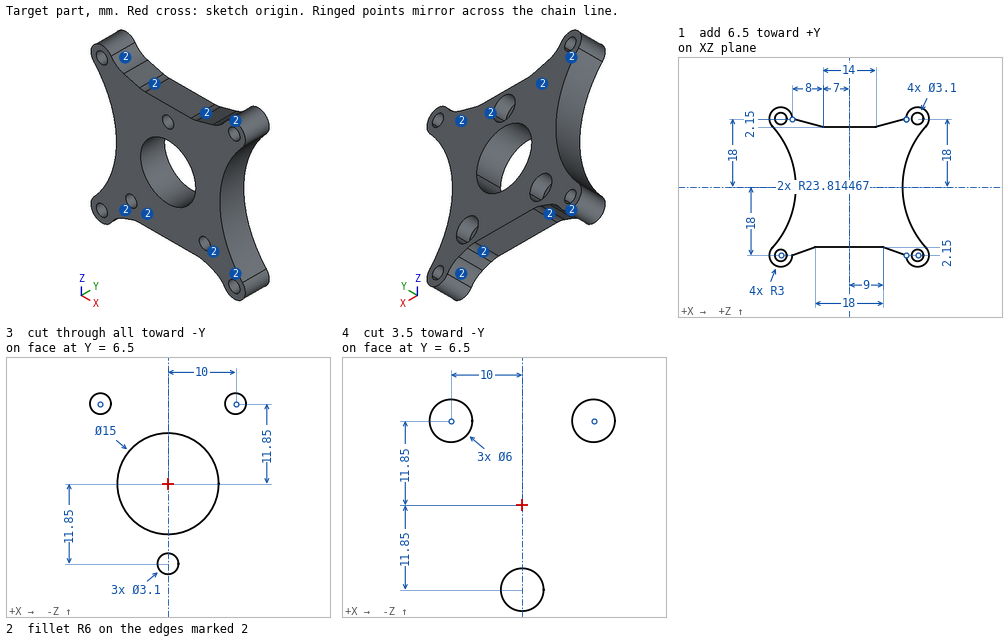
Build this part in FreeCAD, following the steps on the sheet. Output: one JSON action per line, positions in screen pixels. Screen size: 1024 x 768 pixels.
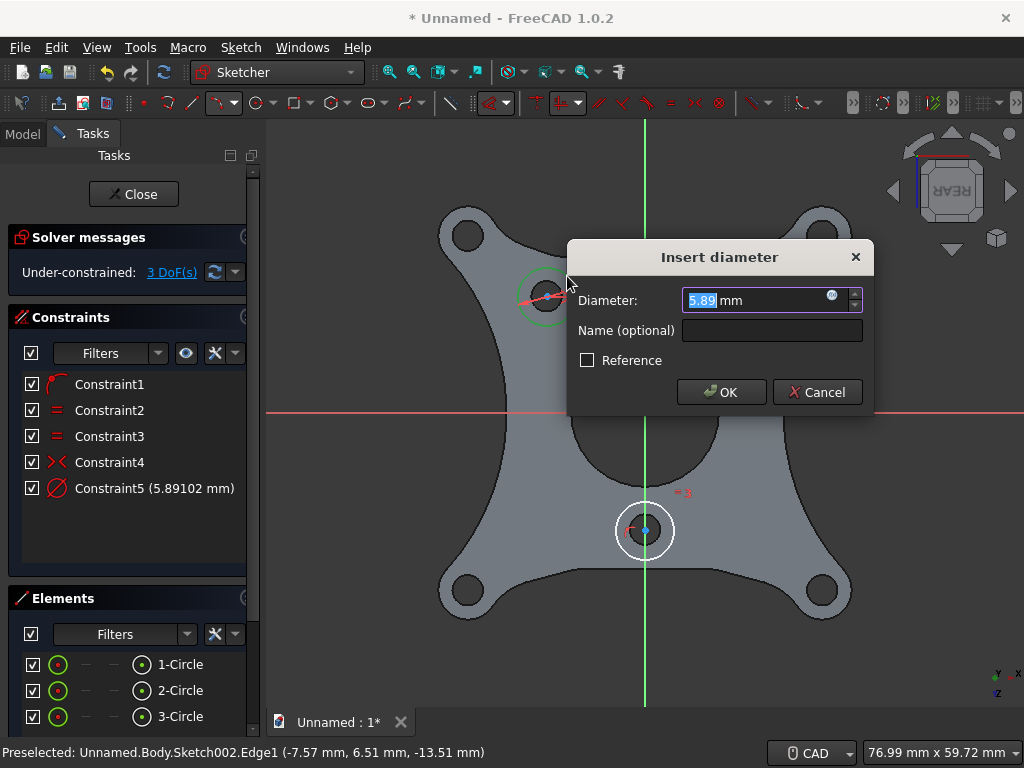
{"action": "type", "text": "6"}
{"action": "key", "text": "Return"}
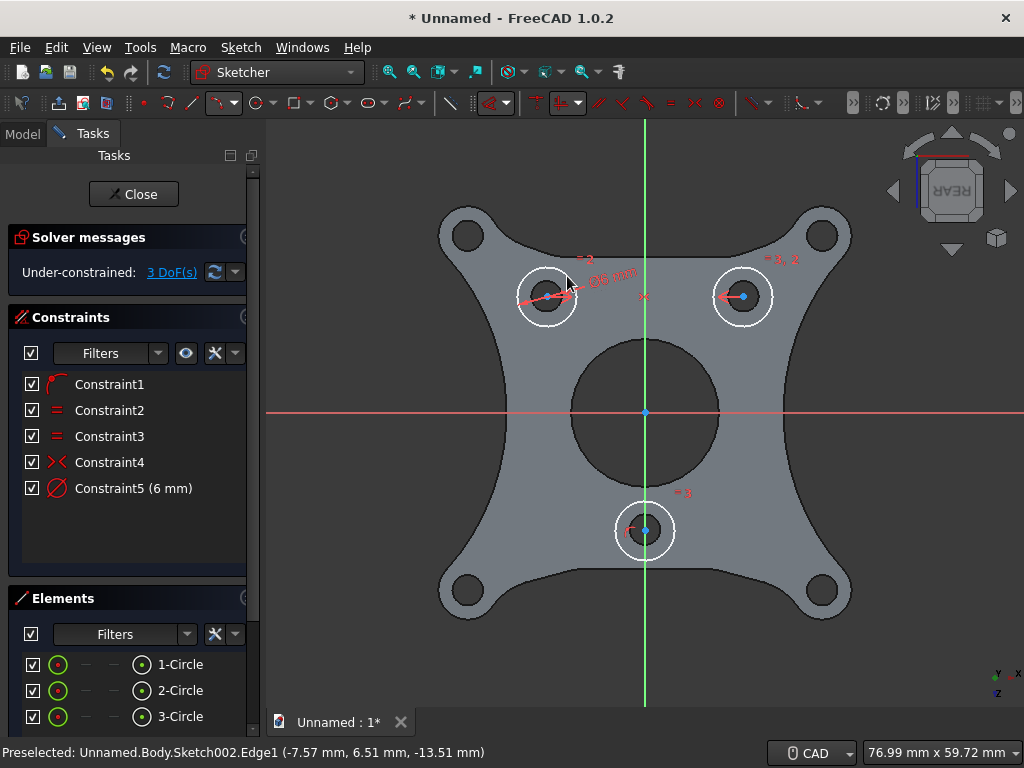
{"action": "left_click", "coordinate": [547, 297]}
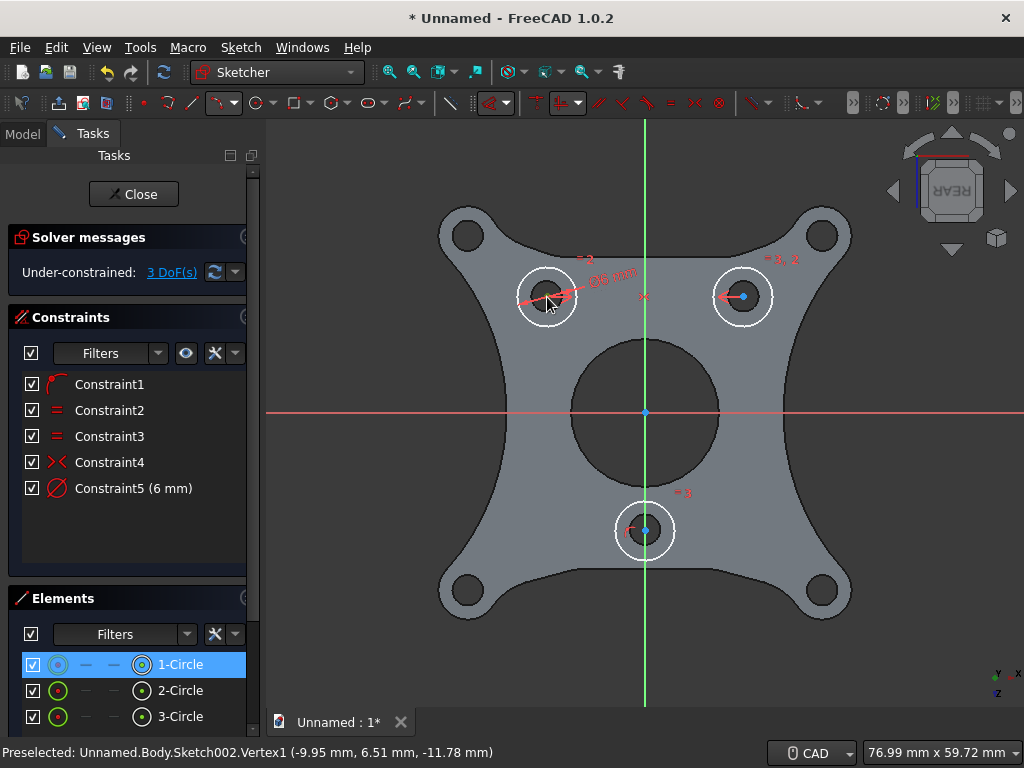
{"action": "left_click", "coordinate": [508, 104]}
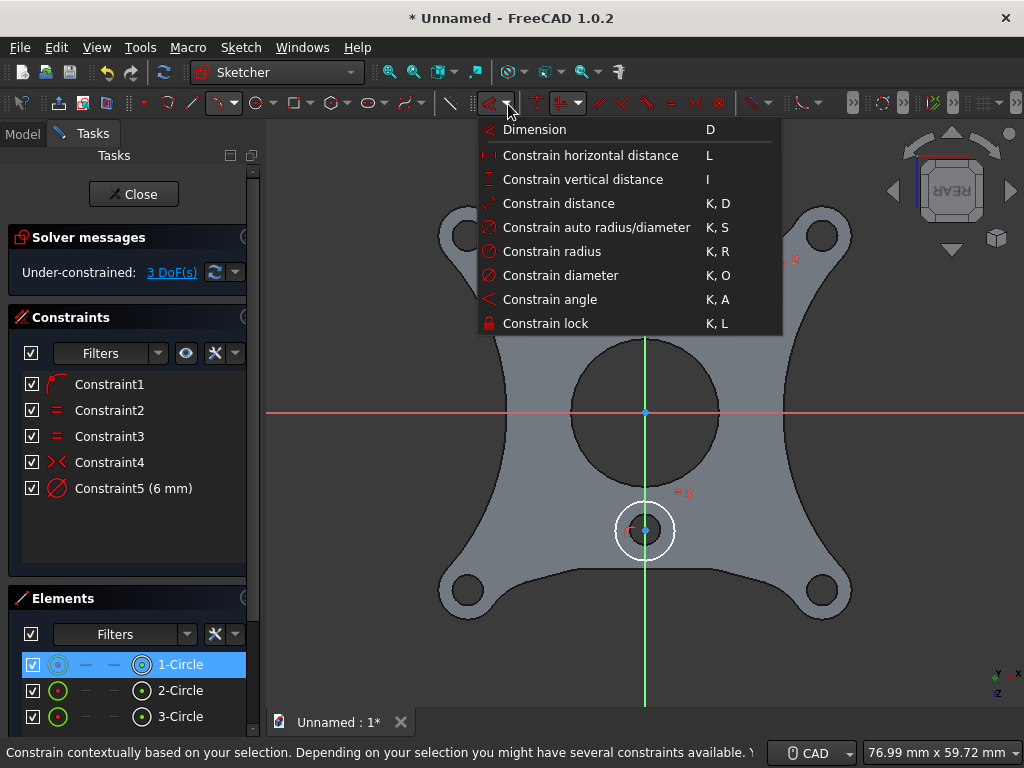
{"action": "left_click", "coordinate": [630, 155]}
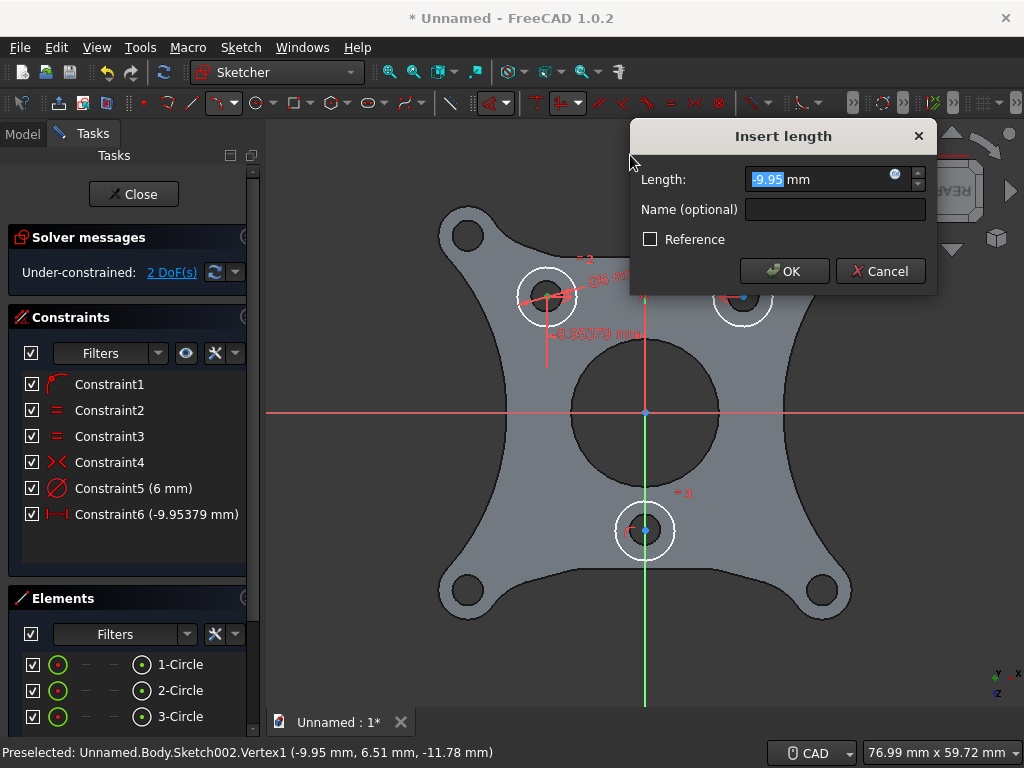
{"action": "type", "text": "-10"}
{"action": "key", "text": "Return"}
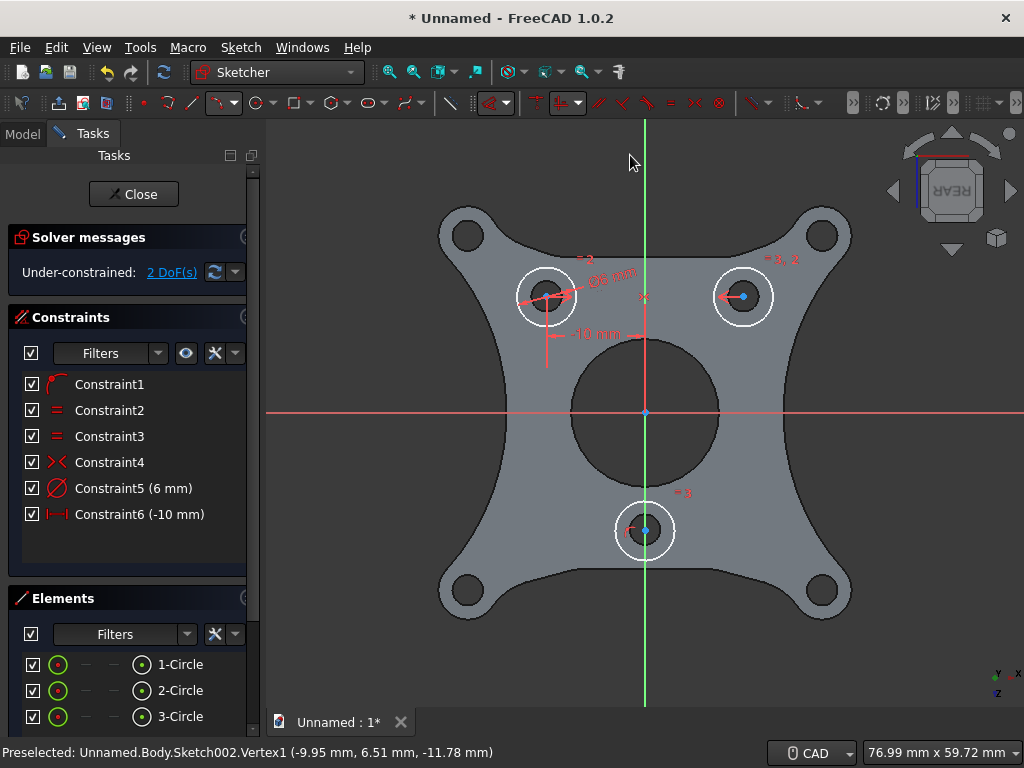
{"action": "left_click", "coordinate": [547, 297]}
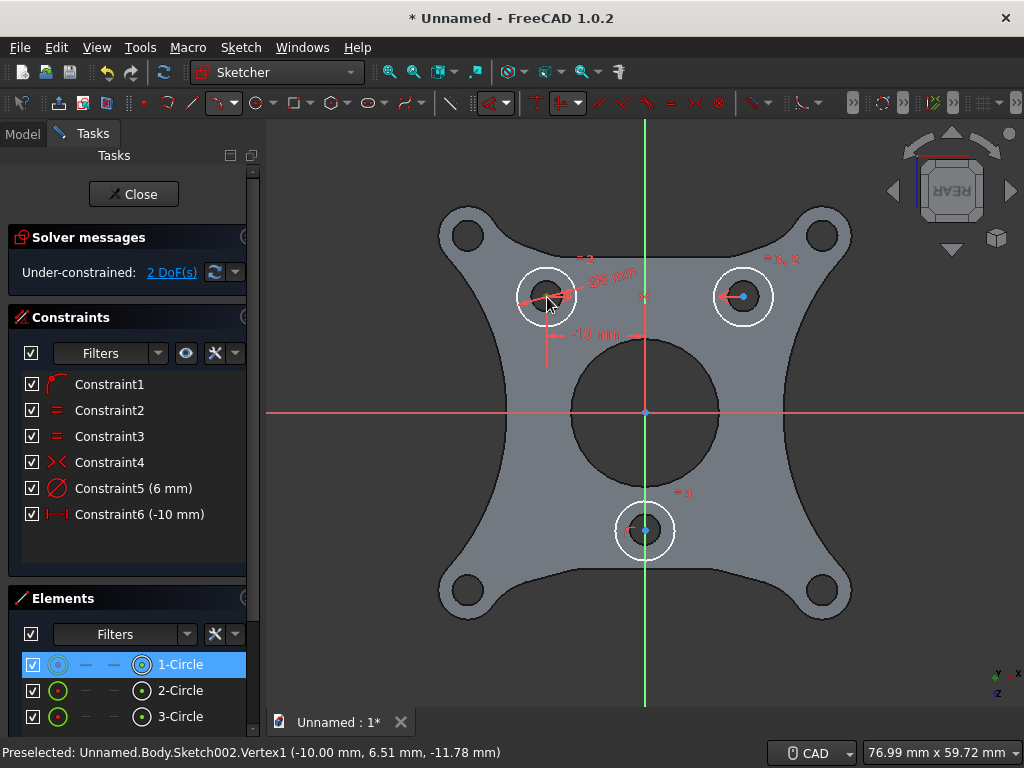
{"action": "left_click", "coordinate": [508, 104]}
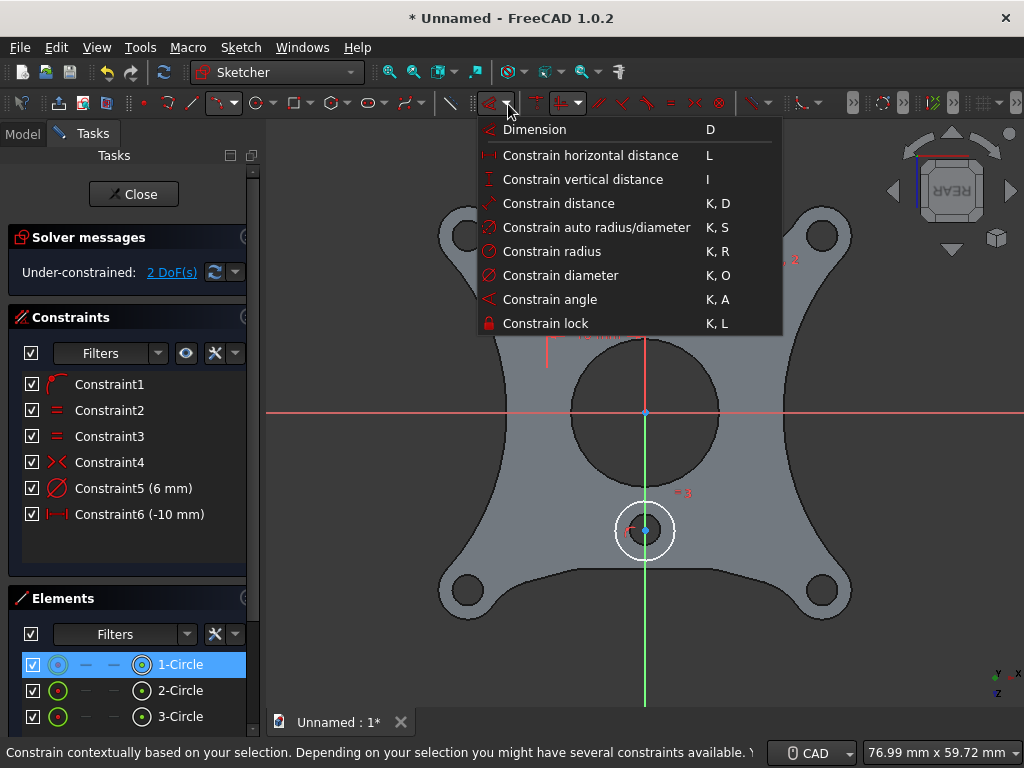
{"action": "left_click", "coordinate": [630, 179]}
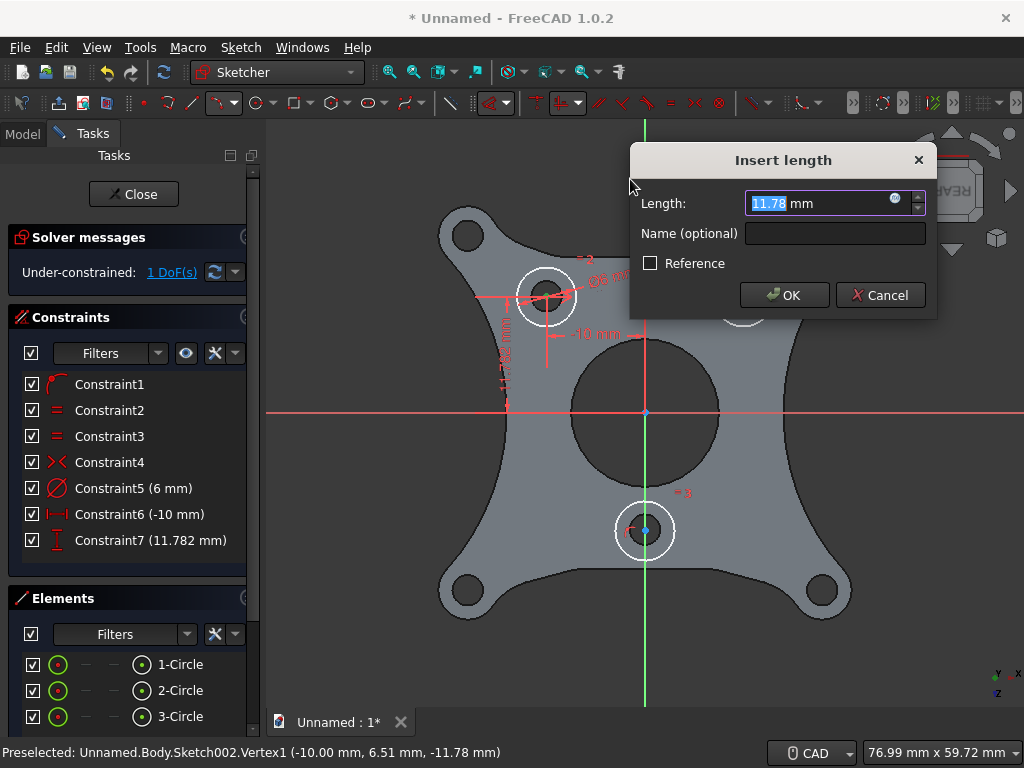
{"action": "type", "text": "11.85"}
{"action": "key", "text": "Return"}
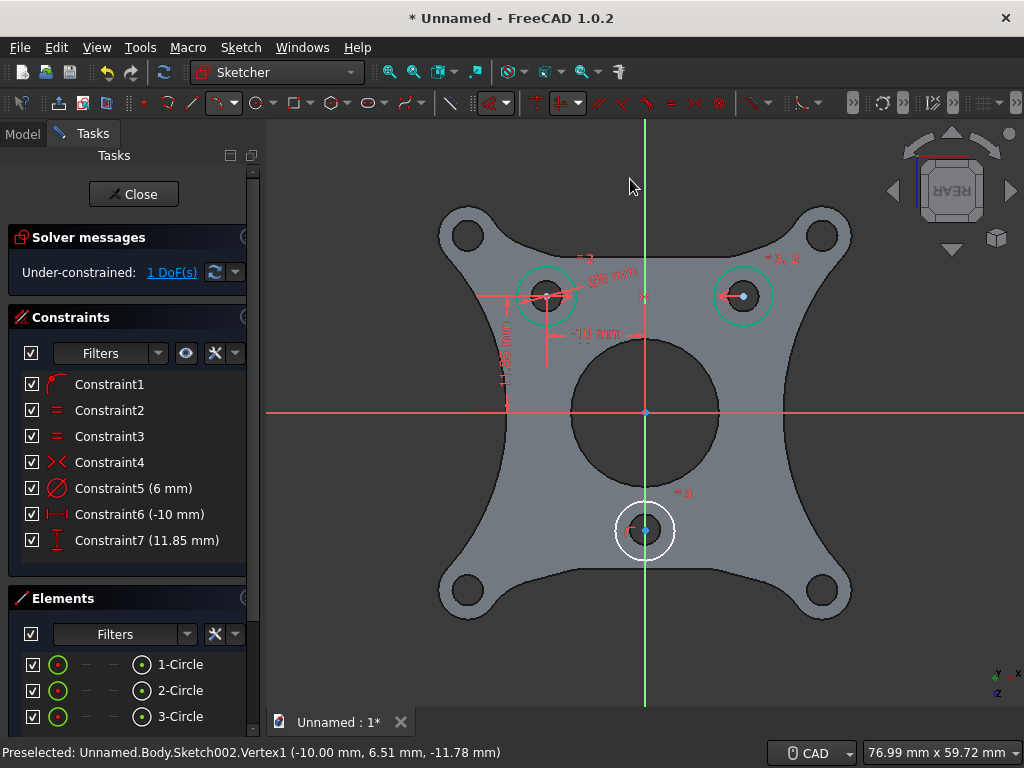
{"action": "left_click", "coordinate": [645, 531]}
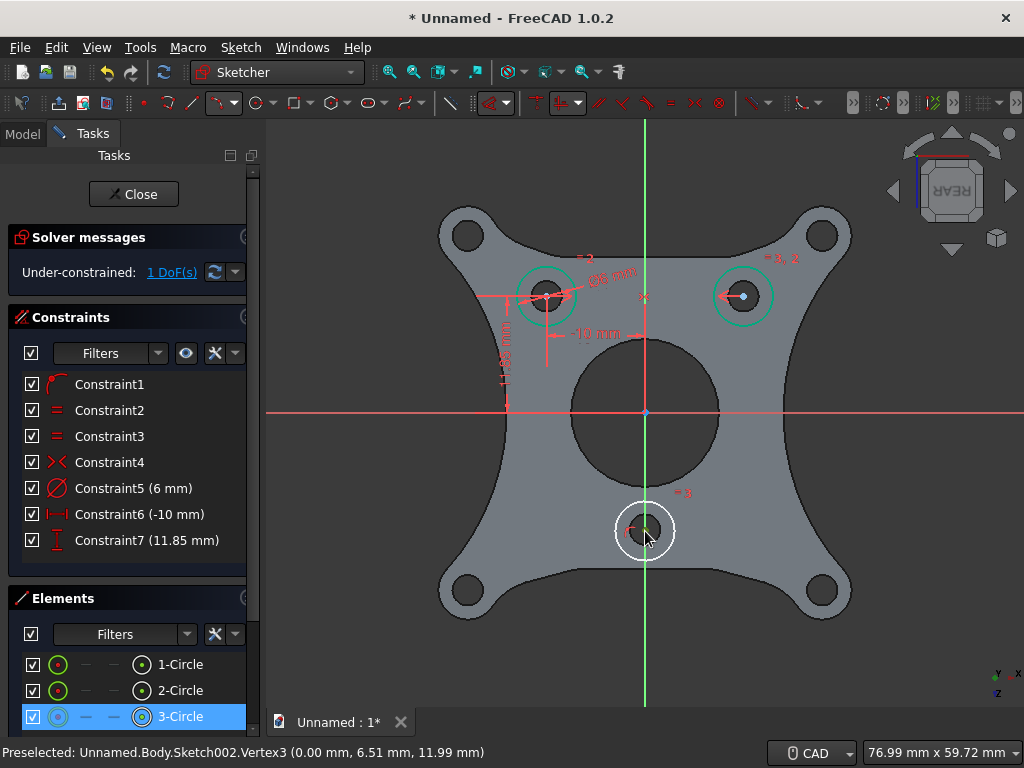
{"action": "key", "text": "i"}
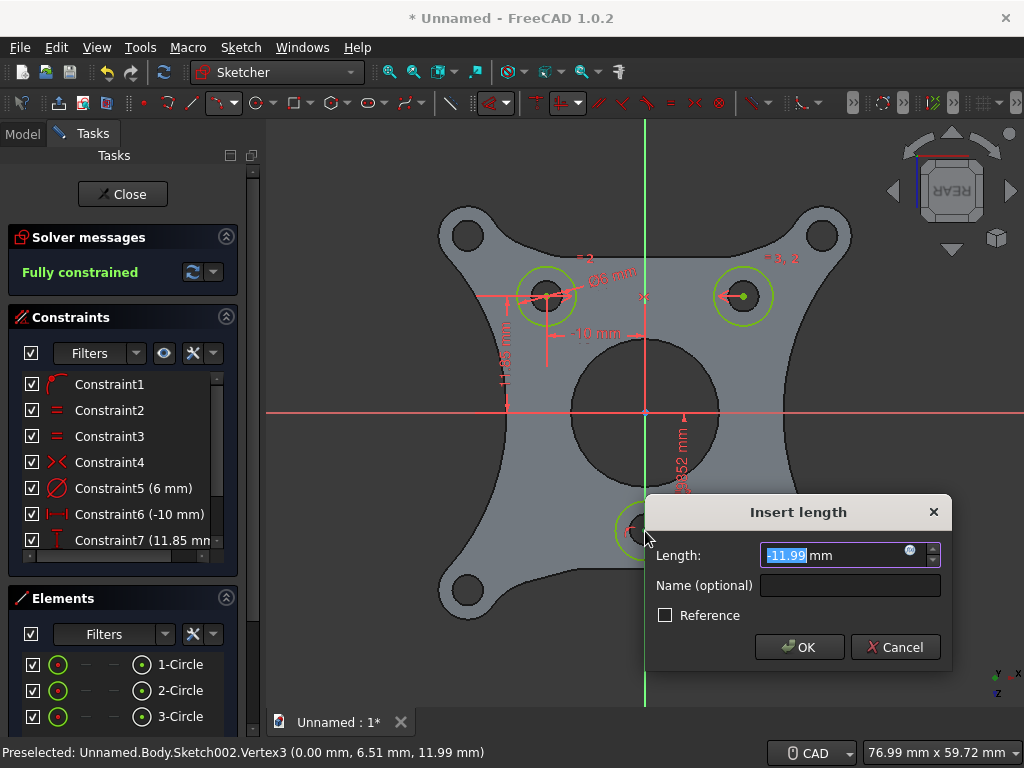
{"action": "type", "text": "-11.85"}
{"action": "key", "text": "Return"}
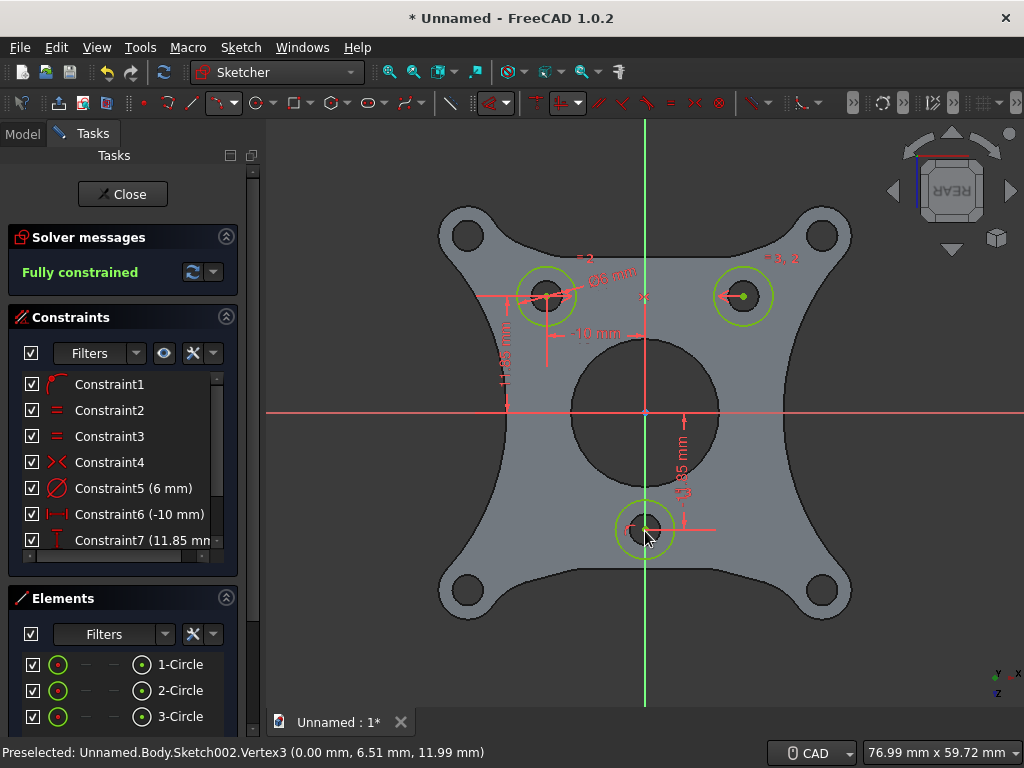
{"action": "left_click", "coordinate": [123, 194]}